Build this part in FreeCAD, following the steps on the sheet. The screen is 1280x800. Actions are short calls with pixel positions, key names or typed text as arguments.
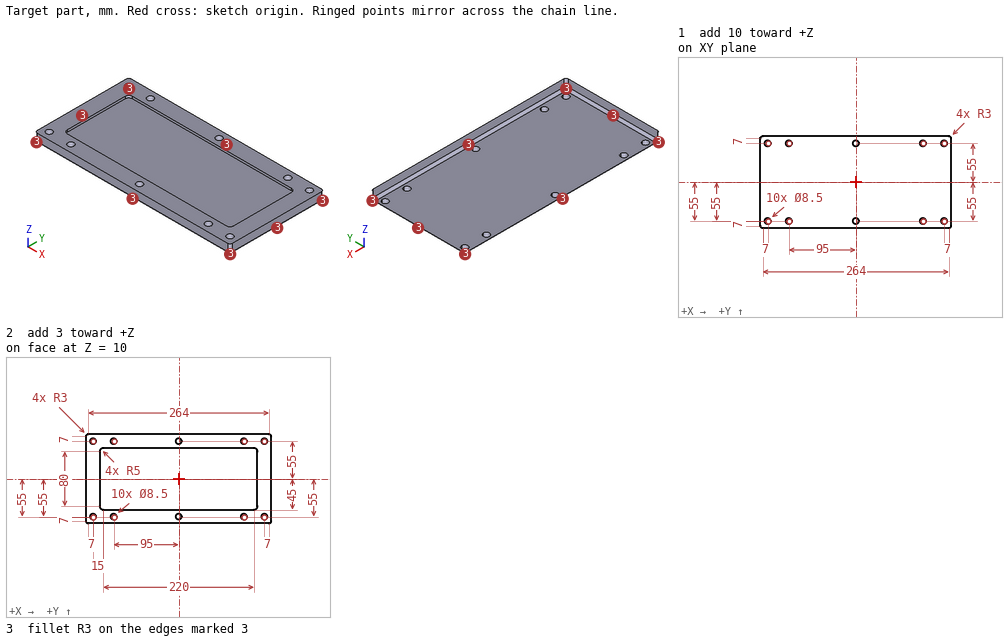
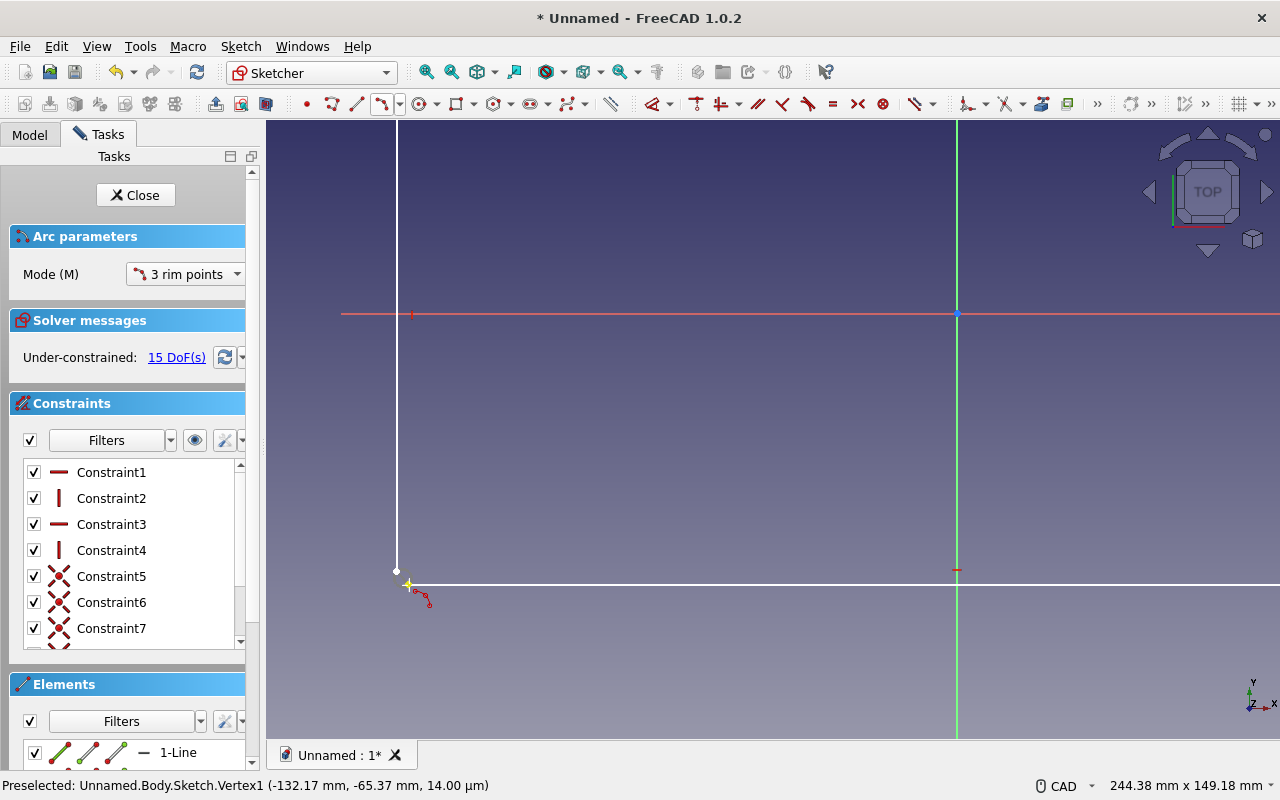
scroll(401, 580, up, 8)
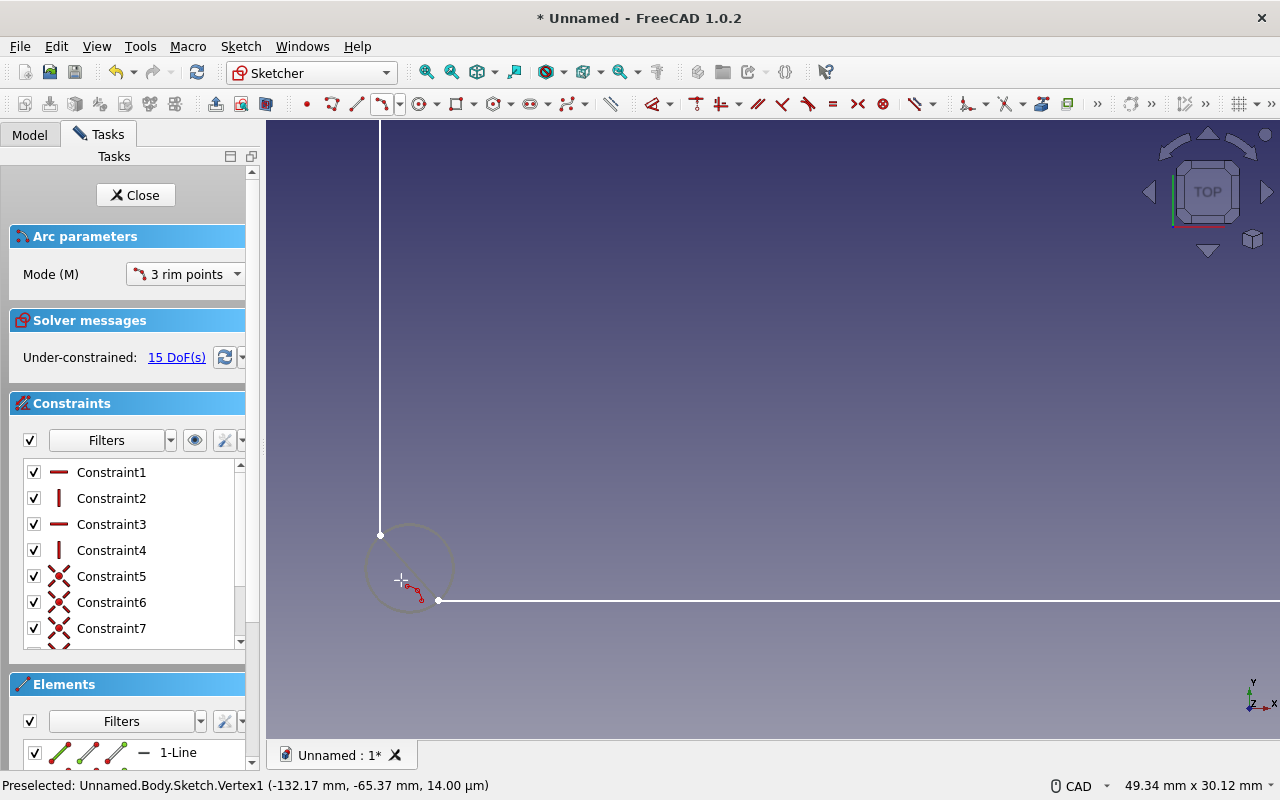
click(399, 575)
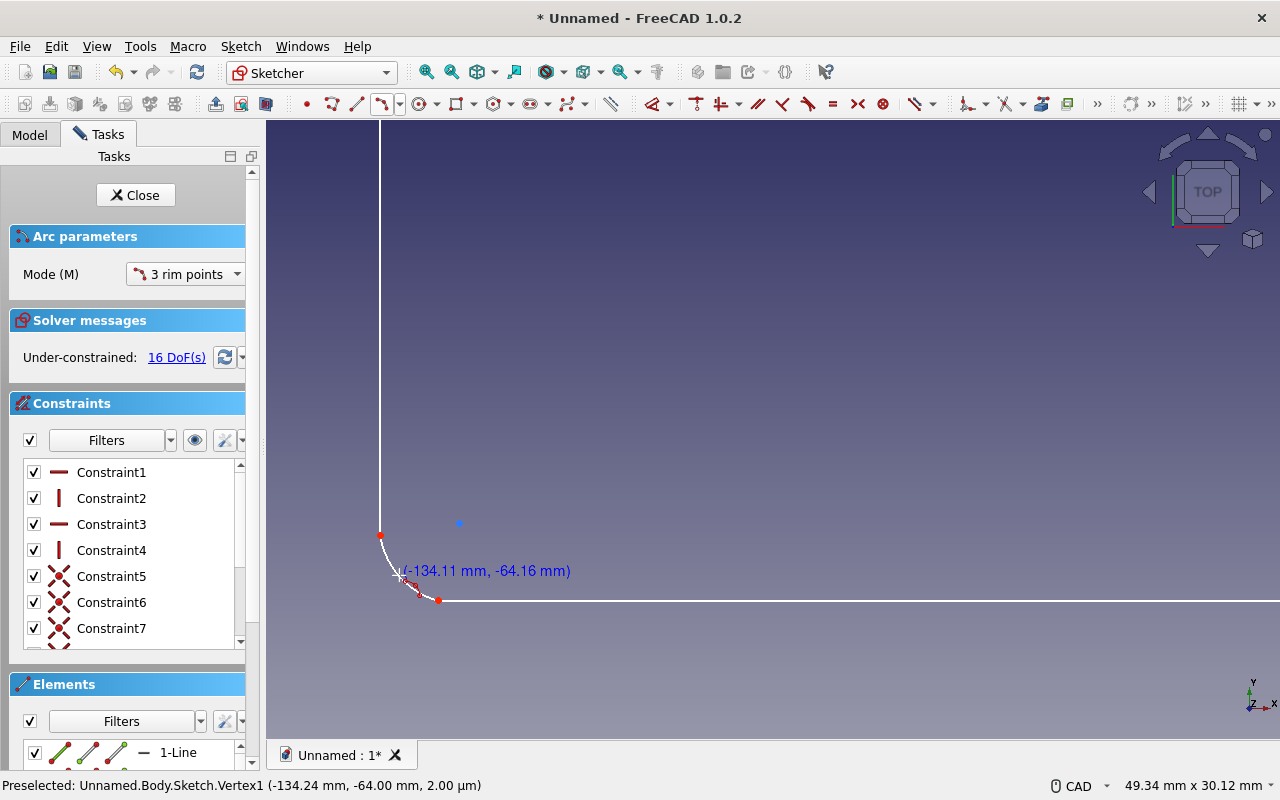
click(418, 104)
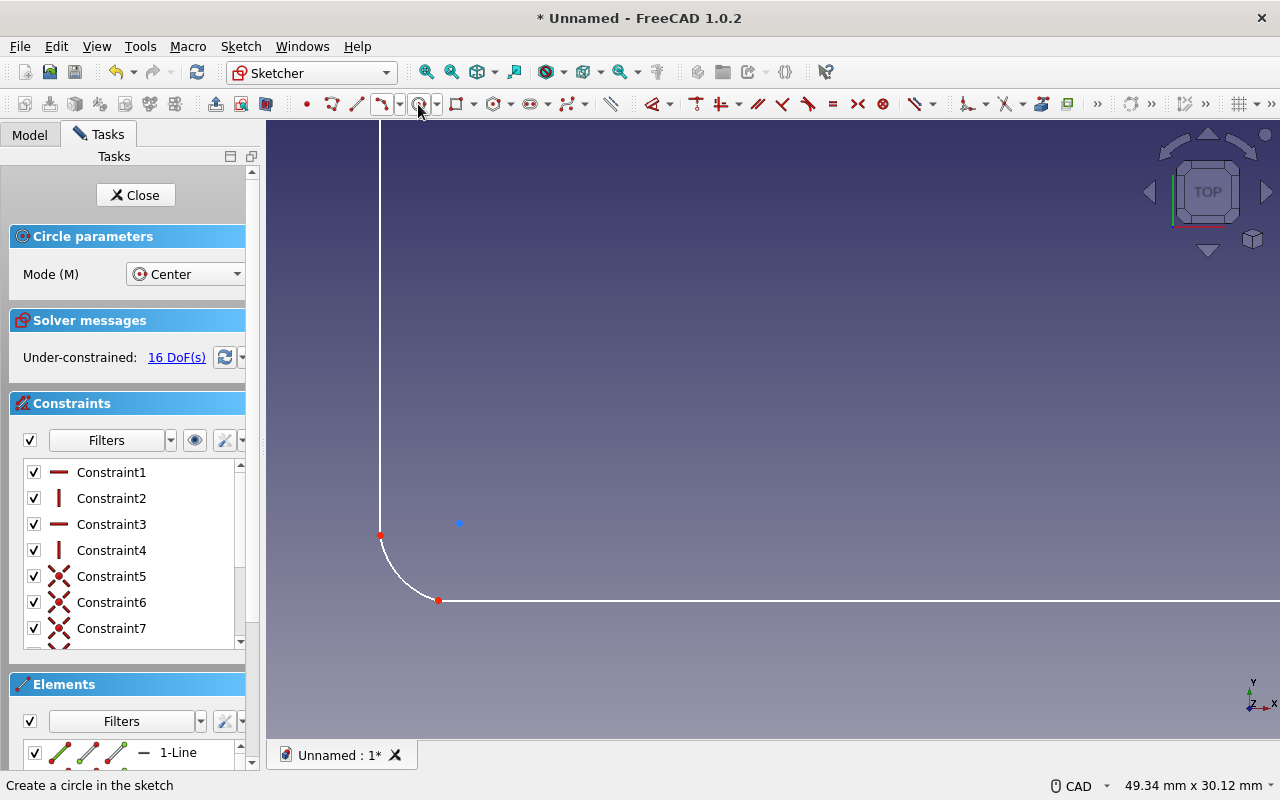
scroll(399, 576, down, 11)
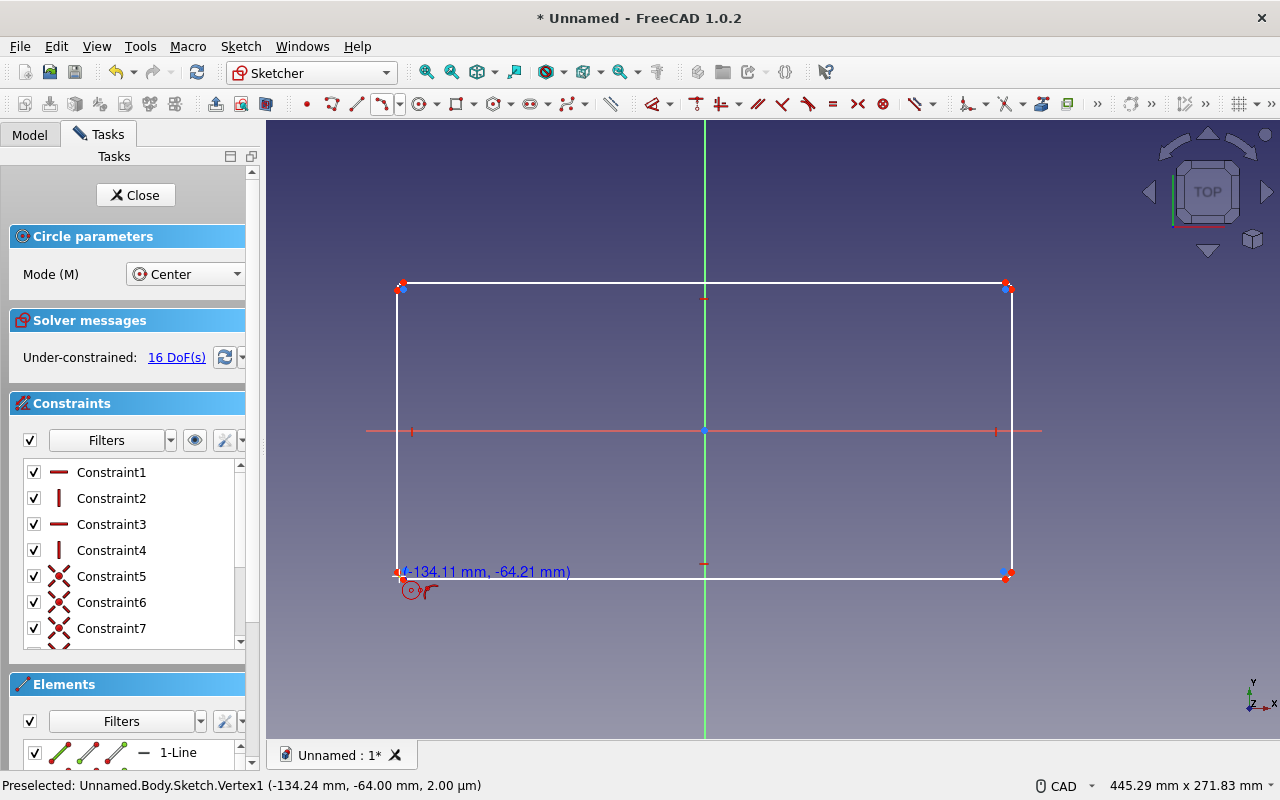
scroll(420, 556, up, 5)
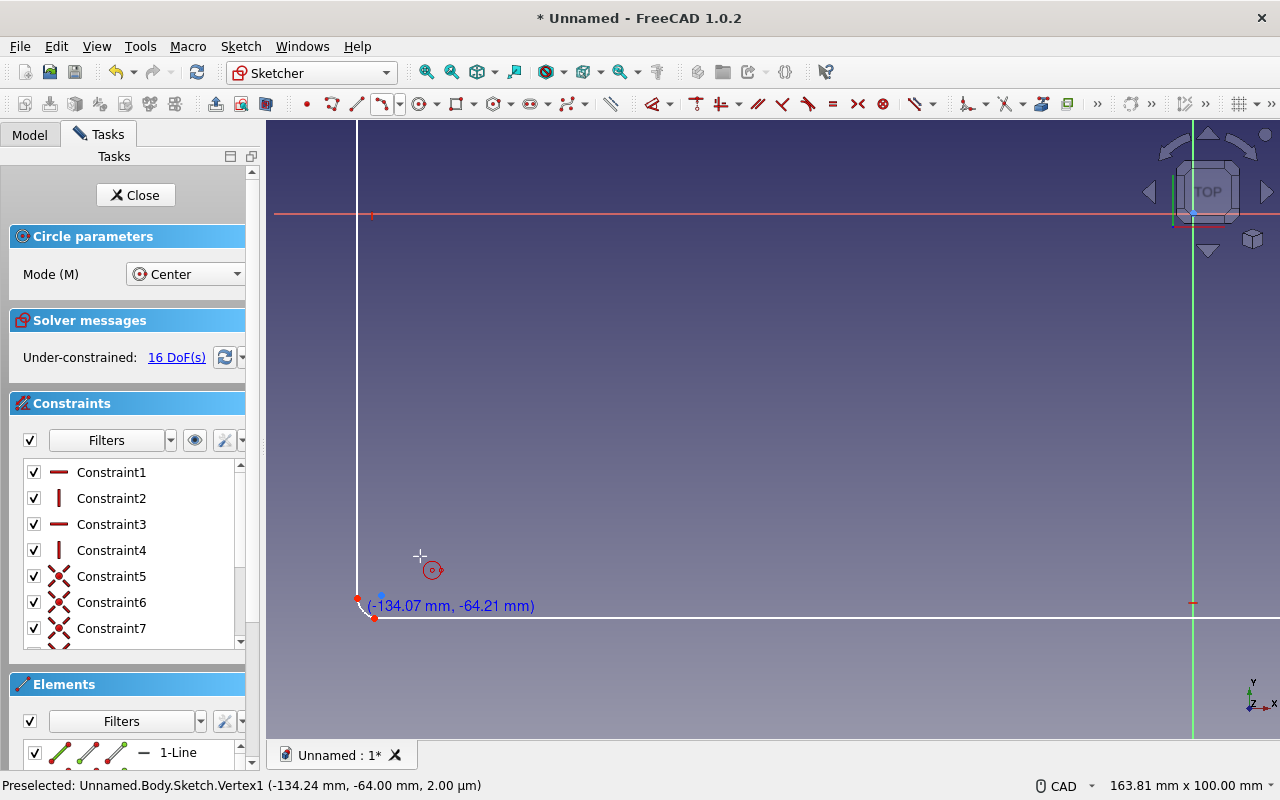
click(419, 554)
move(438, 536)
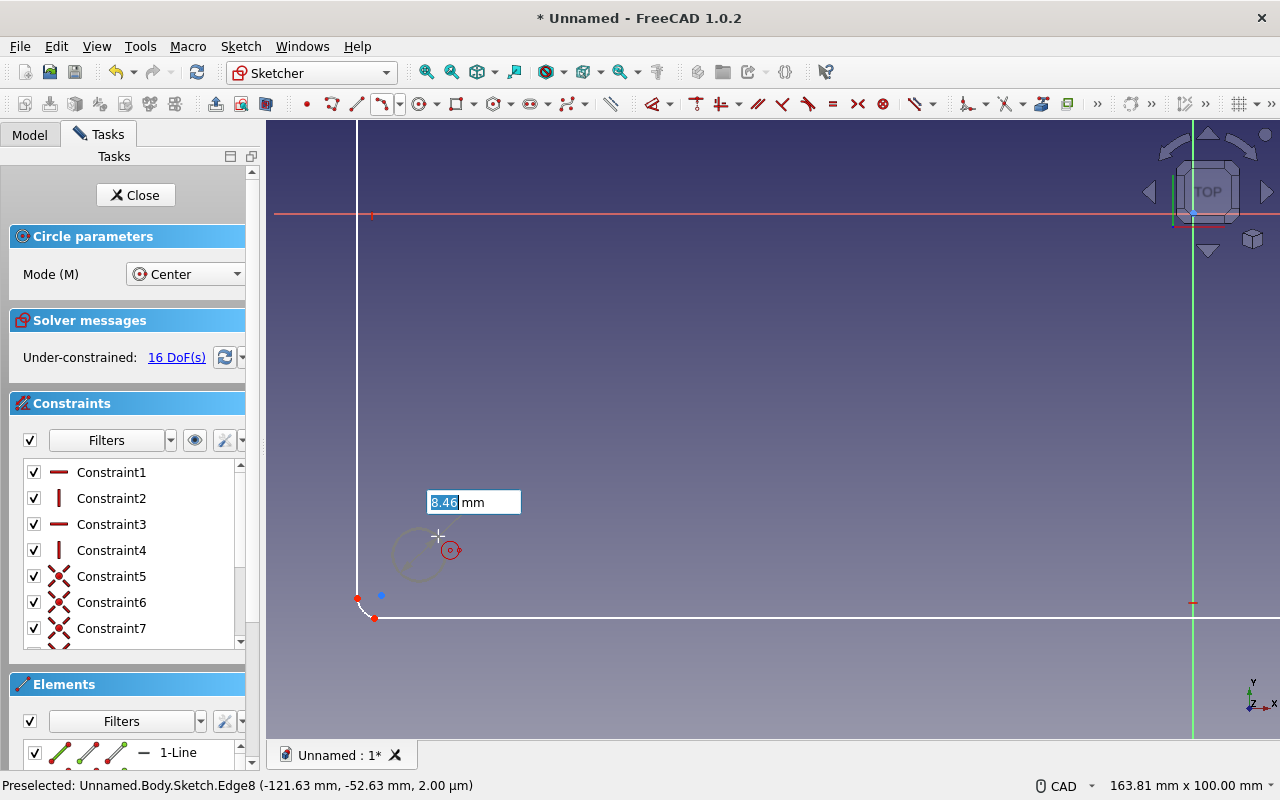
text(8.5)
key(Return)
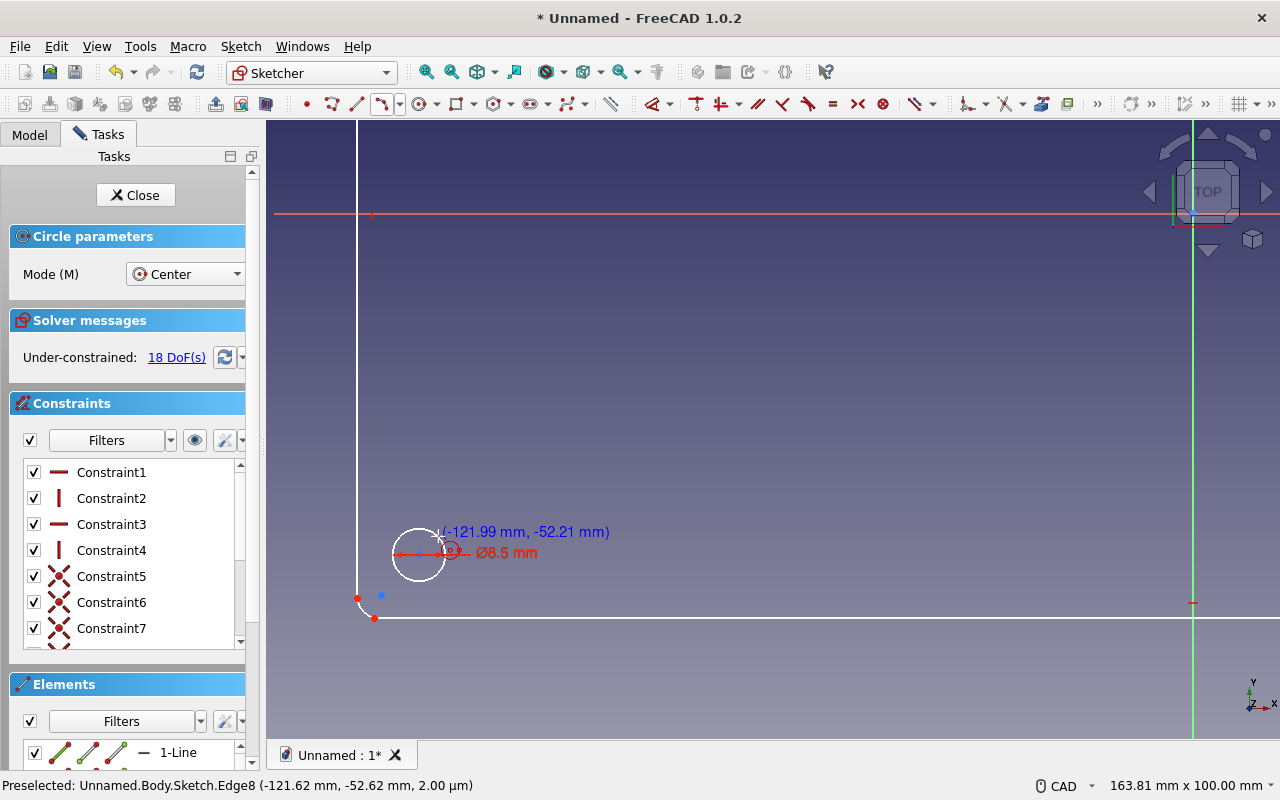
click(605, 554)
move(624, 536)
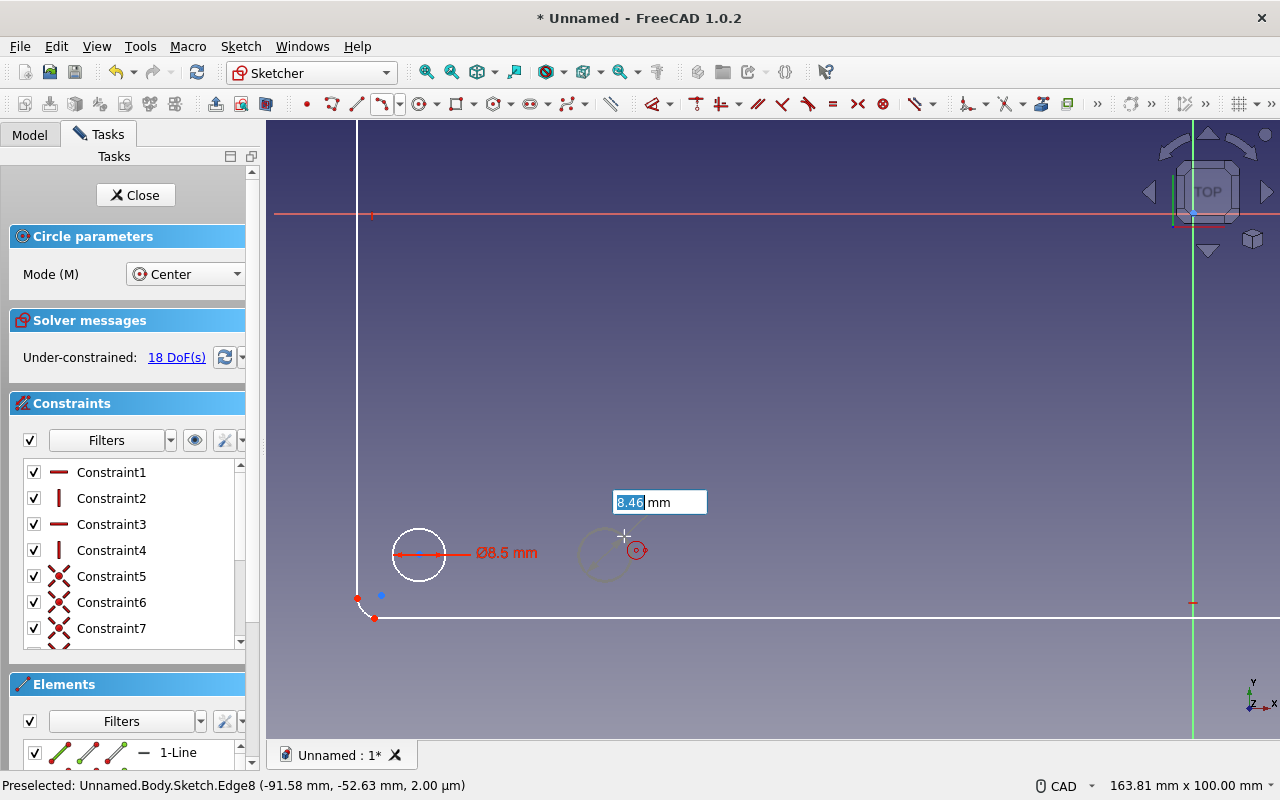
text(8.5)
key(Return)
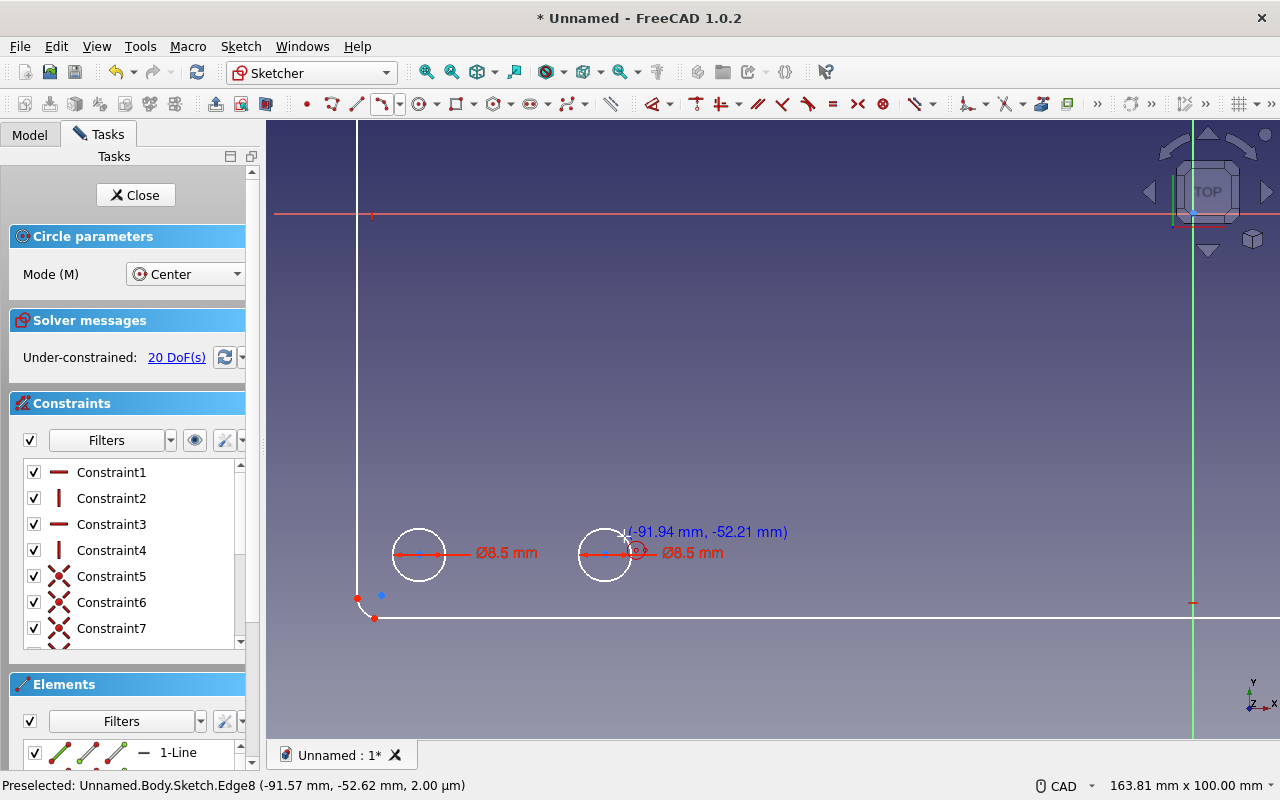
scroll(420, 555, down, 5)